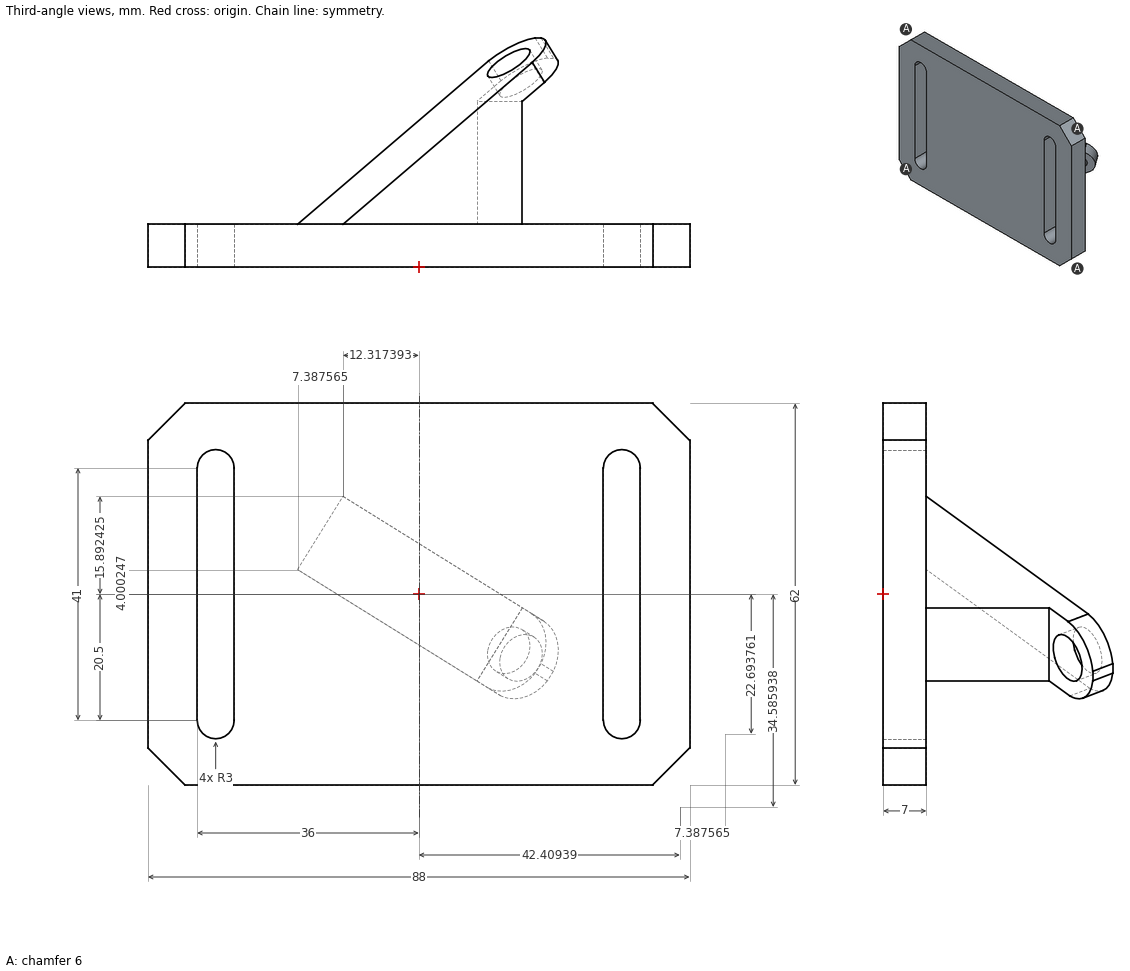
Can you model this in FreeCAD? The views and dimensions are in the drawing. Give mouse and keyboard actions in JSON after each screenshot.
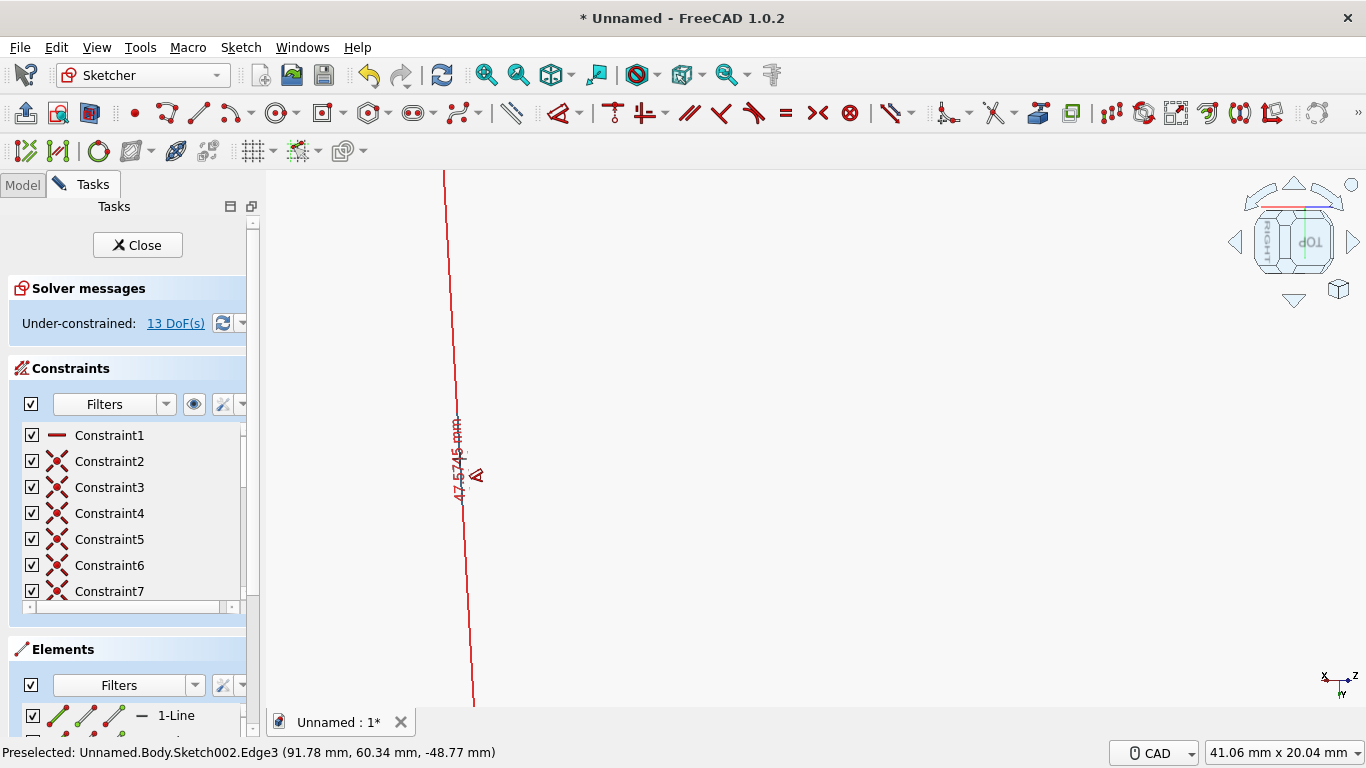
{"action": "key", "text": "Escape"}
{"action": "key", "text": "Escape"}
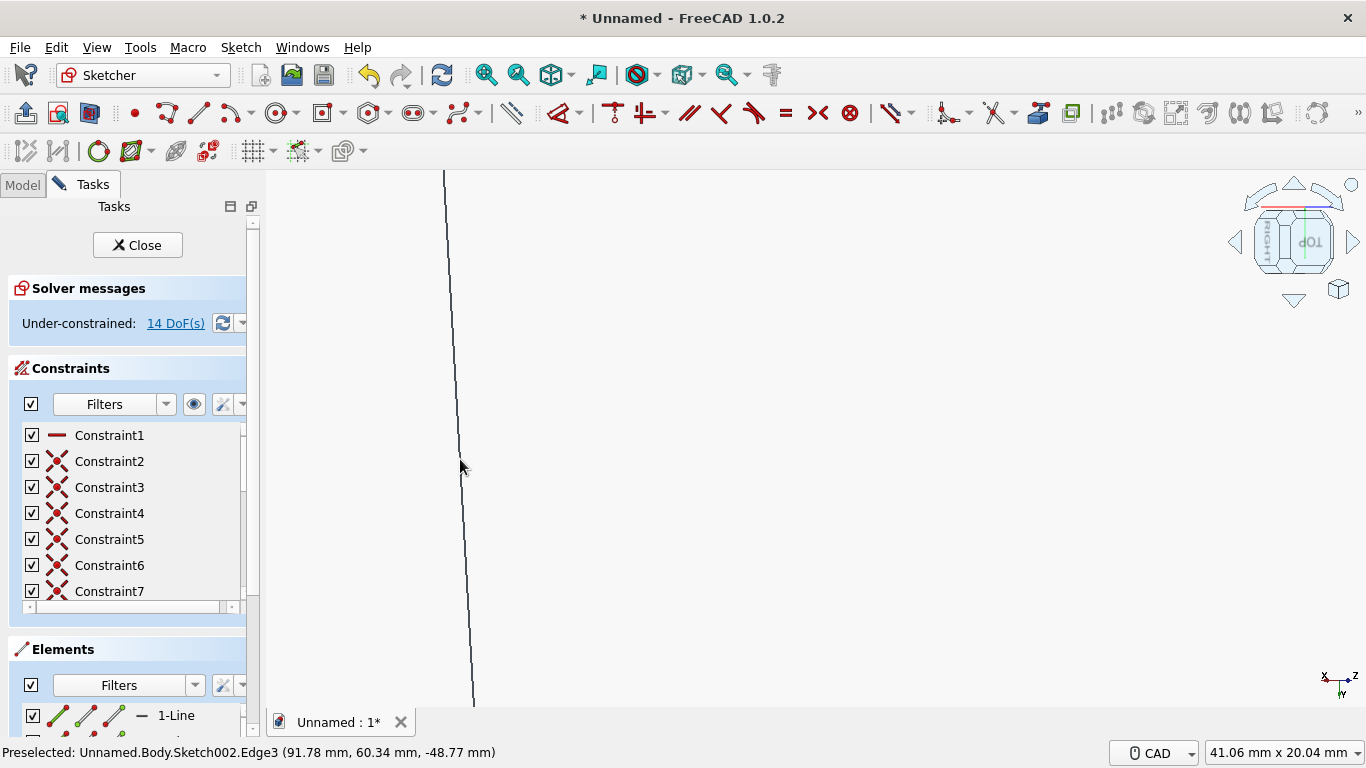
{"action": "left_click", "coordinate": [460, 459]}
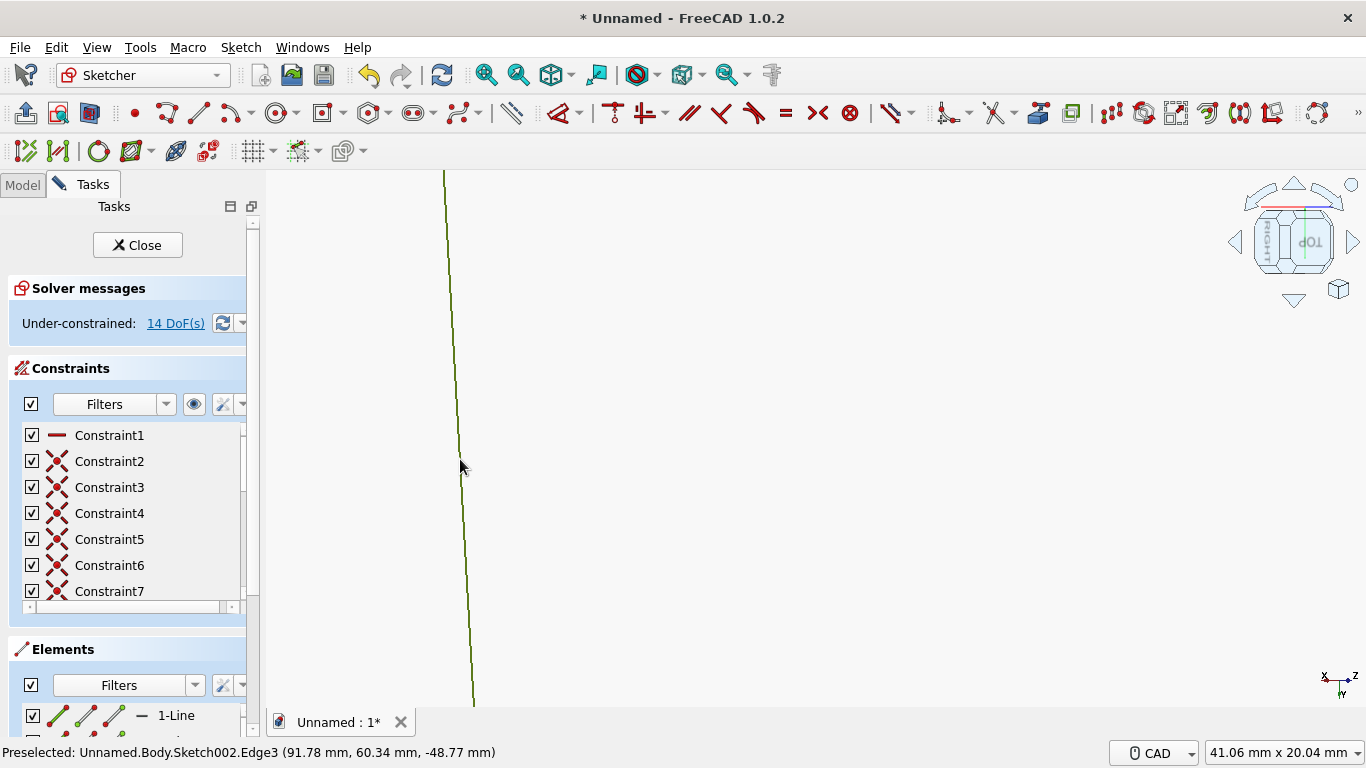
{"action": "left_click", "coordinate": [582, 114]}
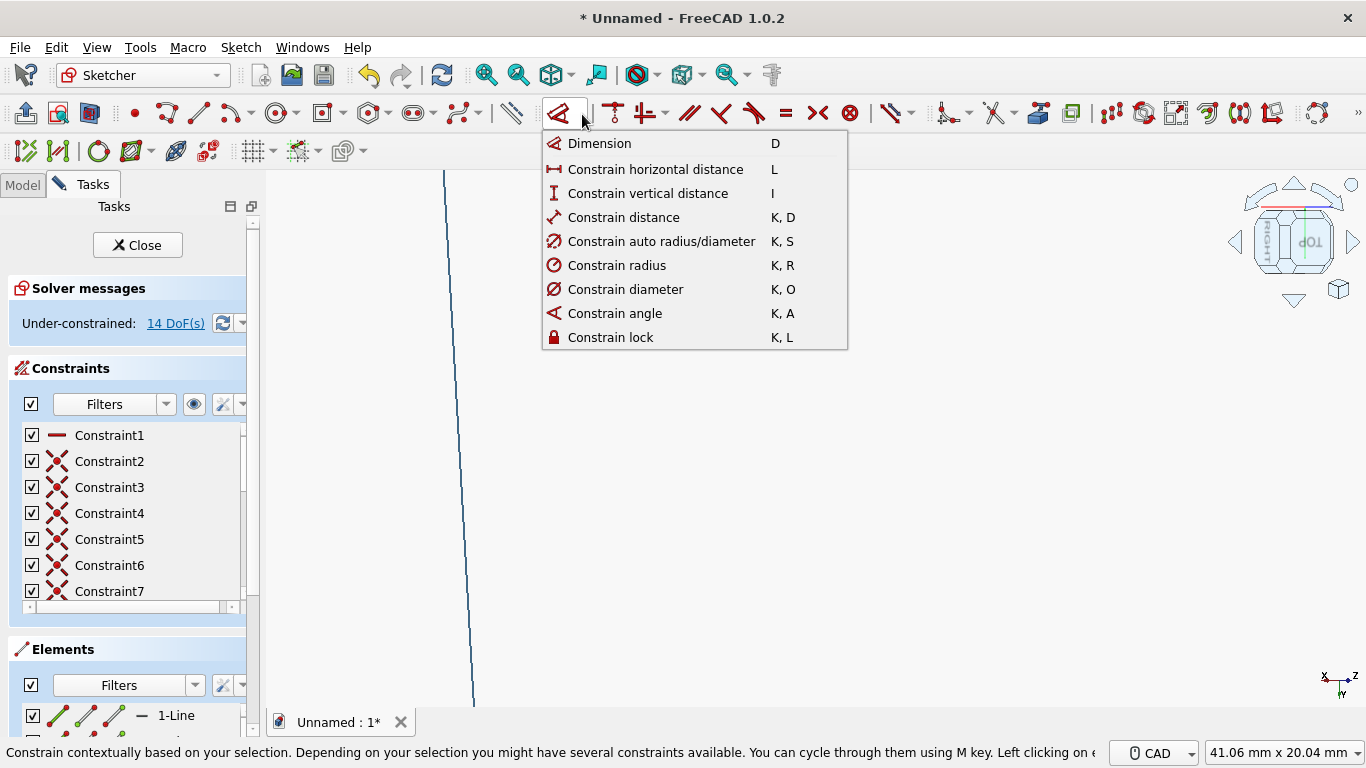
{"action": "left_click", "coordinate": [695, 169]}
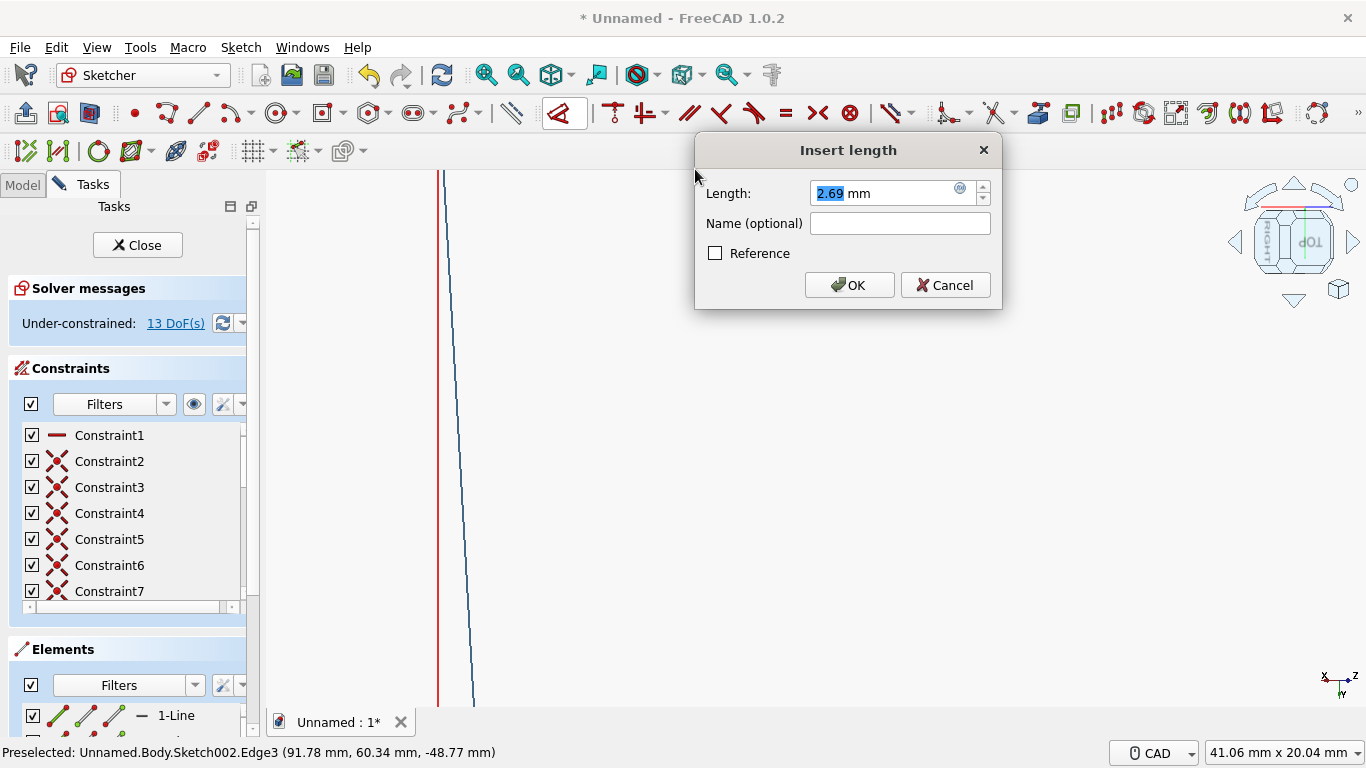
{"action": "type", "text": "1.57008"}
{"action": "key", "text": "Return"}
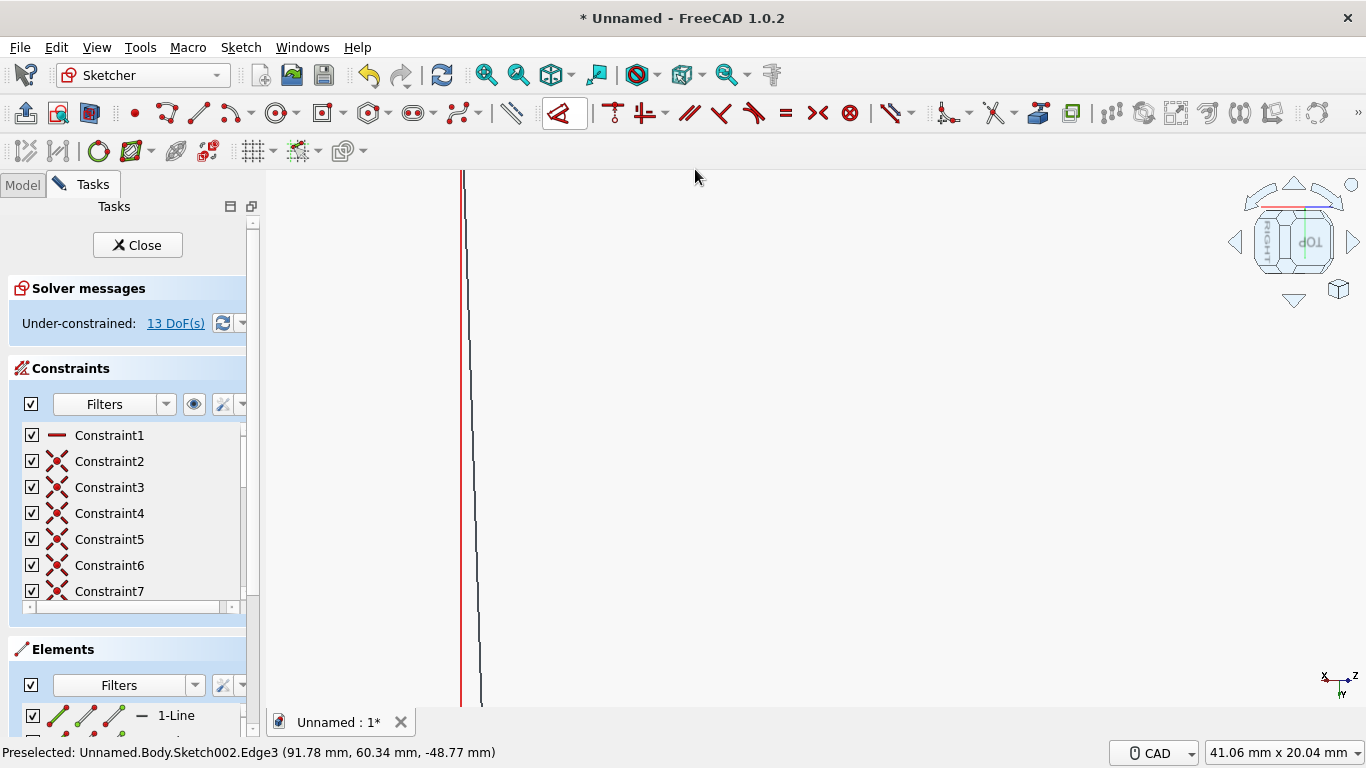
{"action": "scroll", "coordinate": [459, 459], "scroll_direction": "down", "scroll_amount": 11}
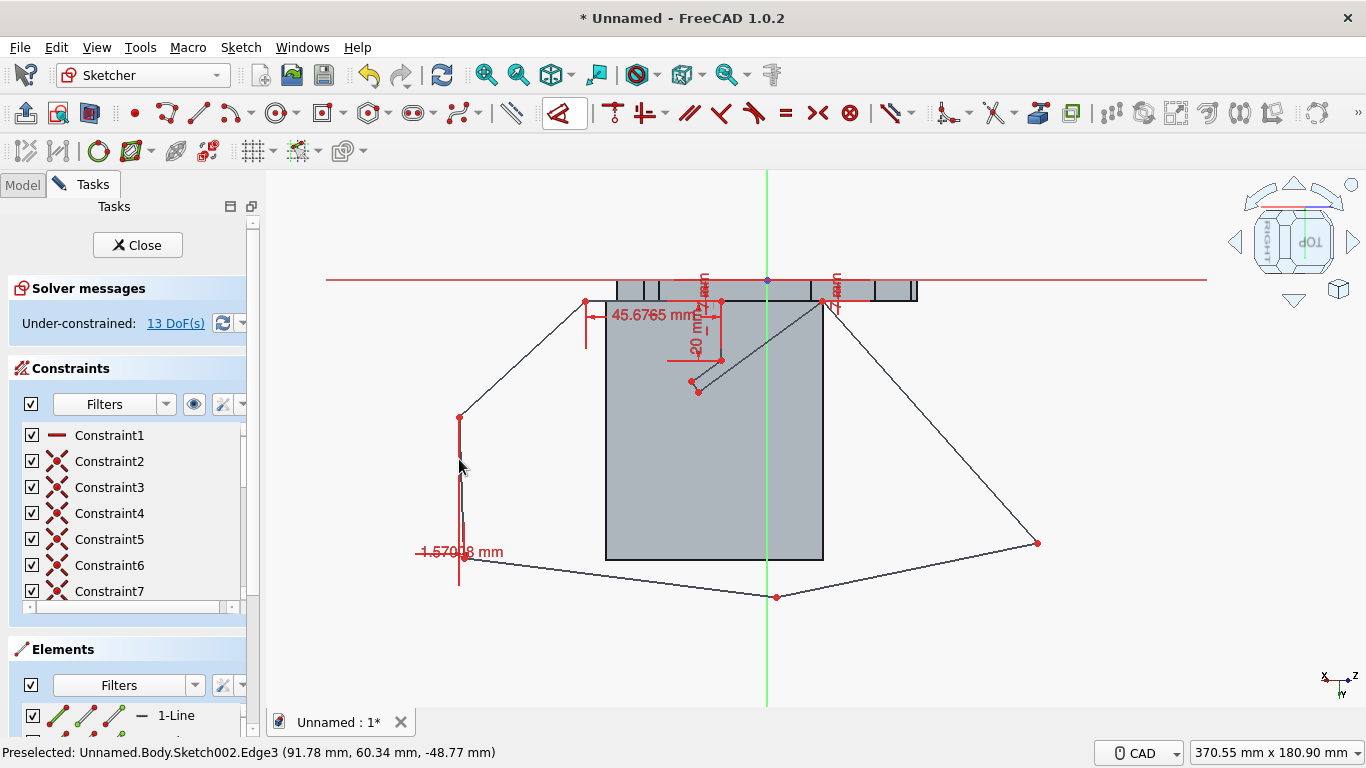
{"action": "scroll", "coordinate": [776, 598], "scroll_direction": "up", "scroll_amount": 8}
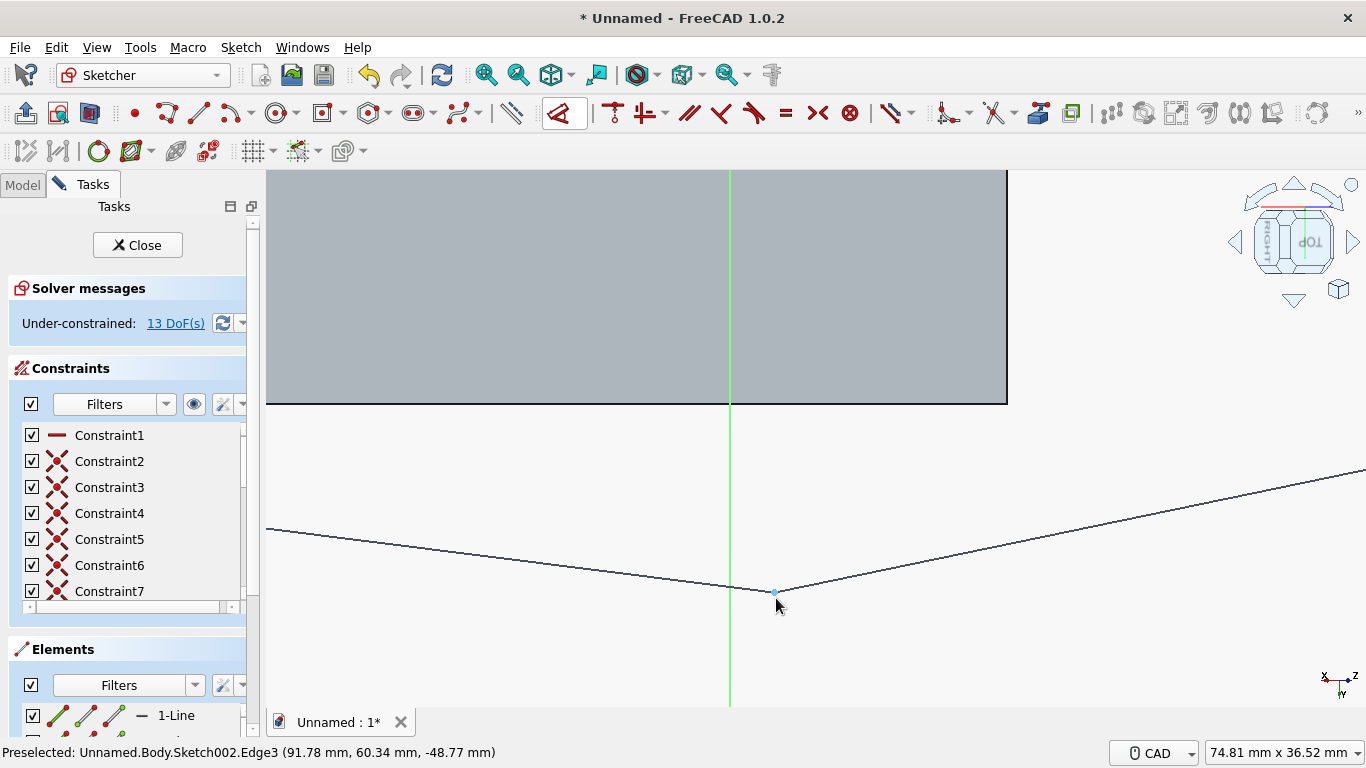
{"action": "left_click", "coordinate": [775, 593]}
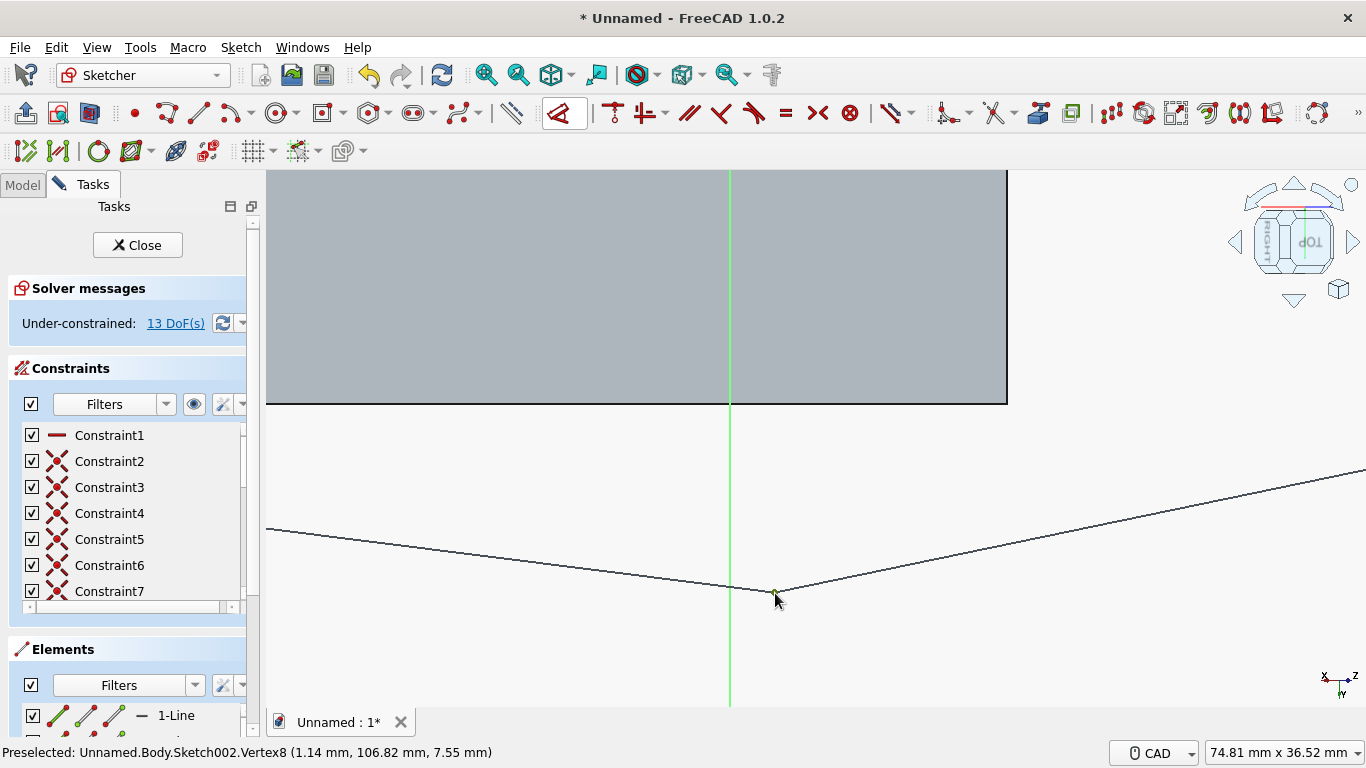
{"action": "key", "text": "l"}